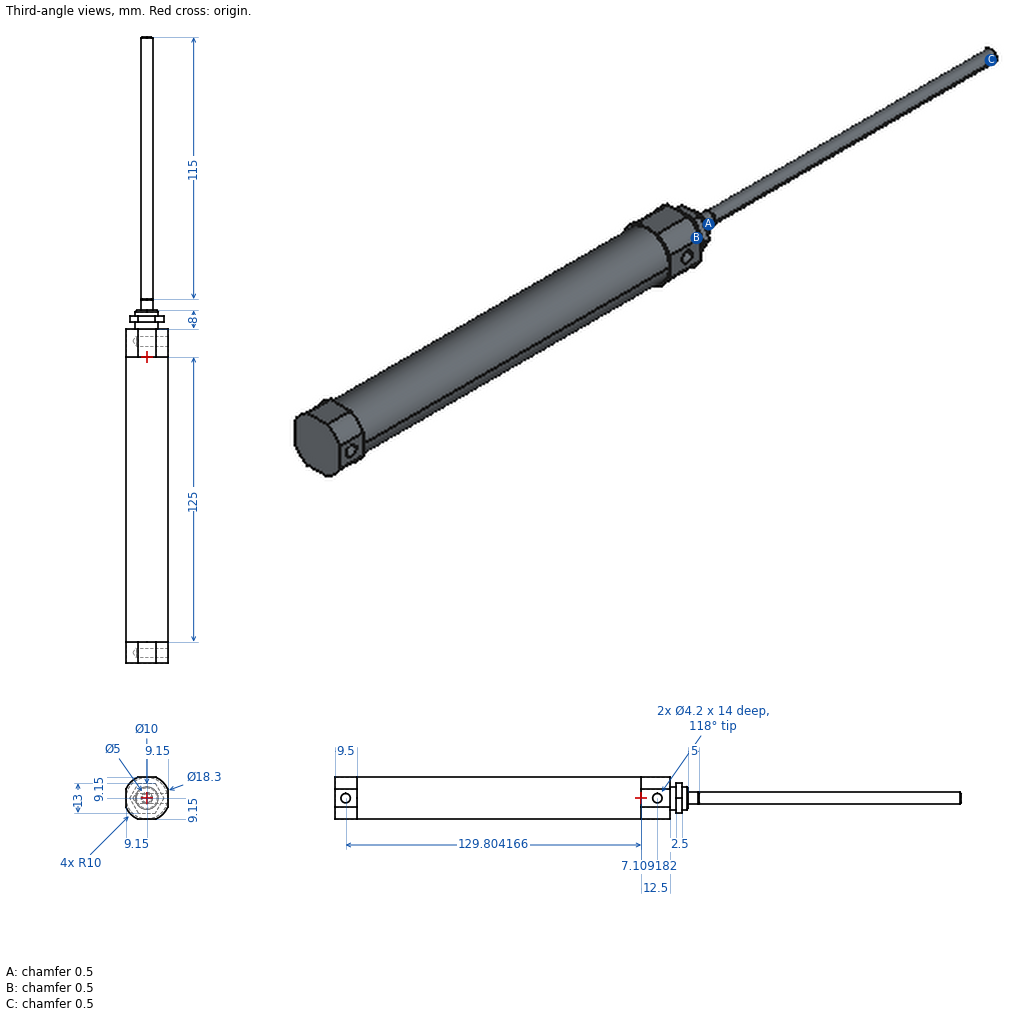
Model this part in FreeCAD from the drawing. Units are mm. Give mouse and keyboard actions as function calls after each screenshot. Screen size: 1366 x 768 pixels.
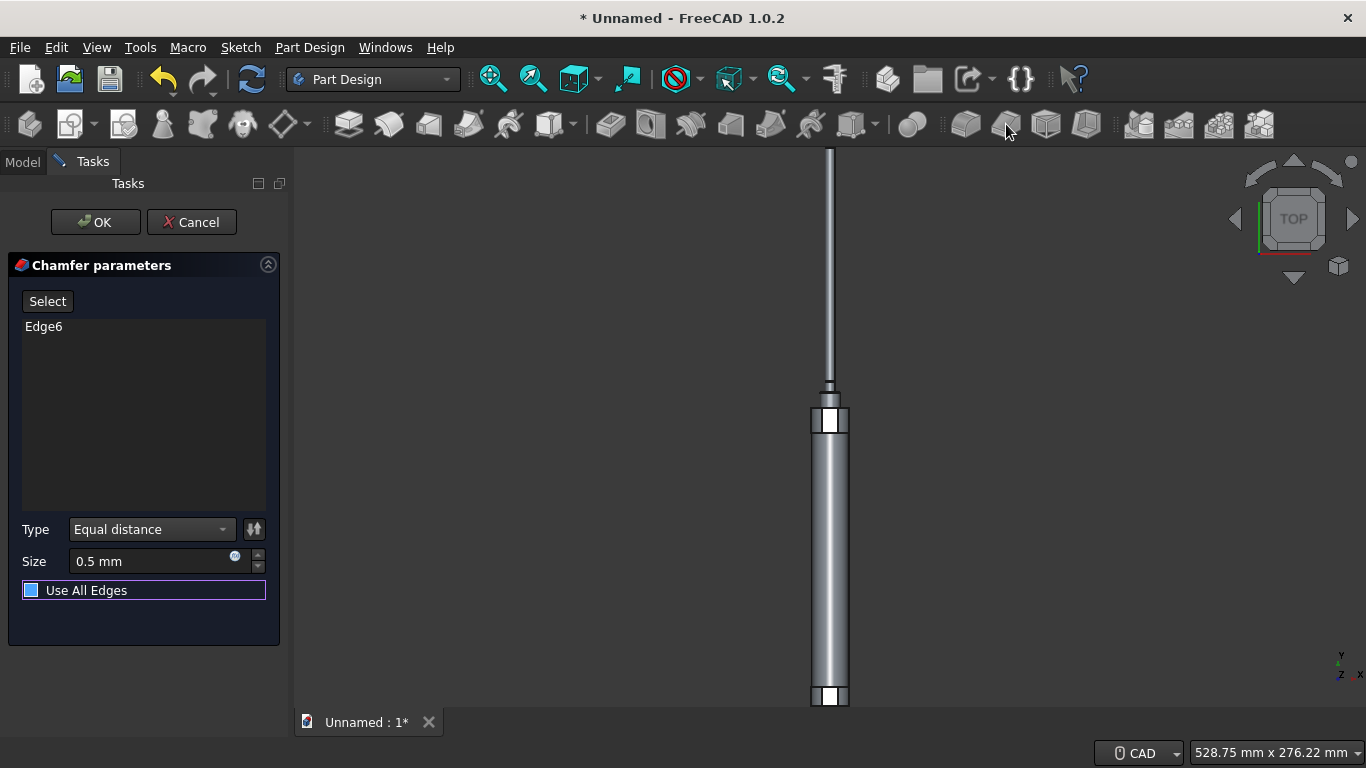
click(96, 222)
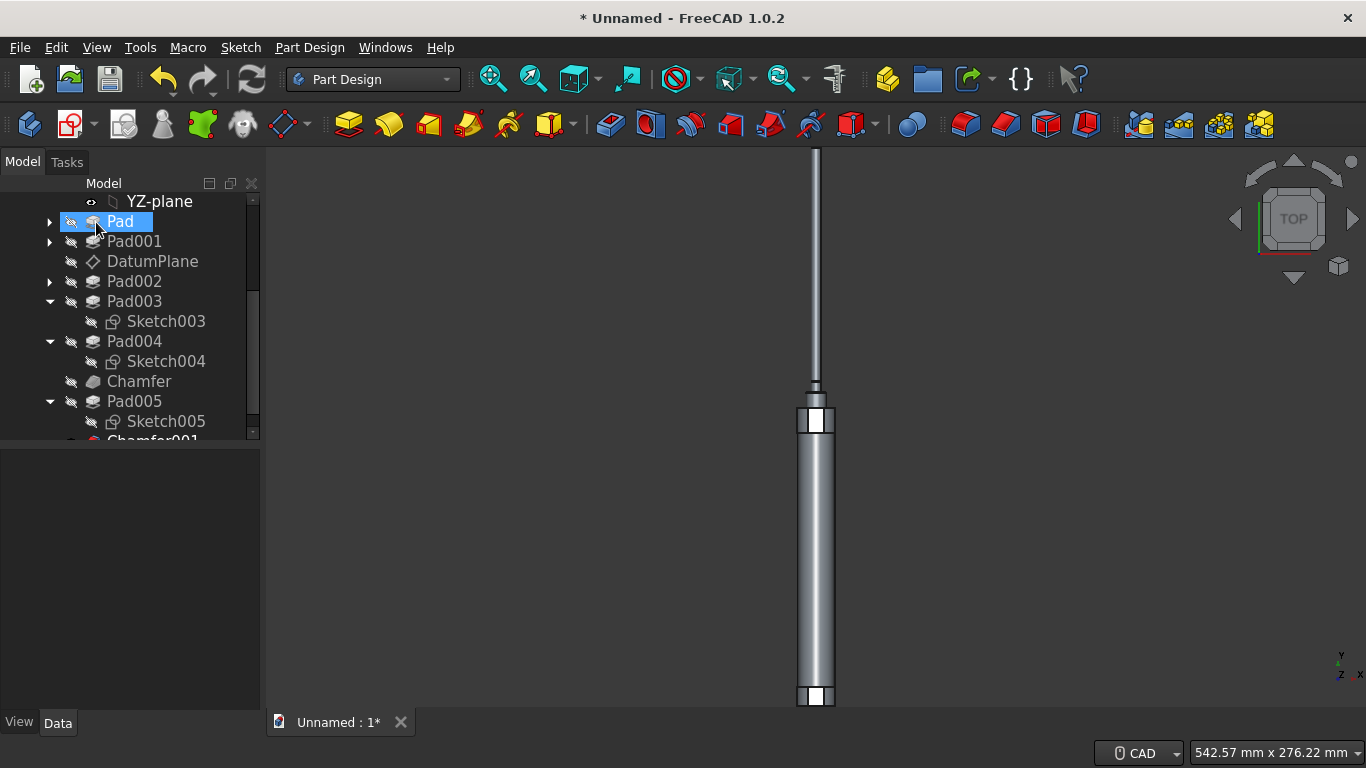
scroll(160, 317, down, 3)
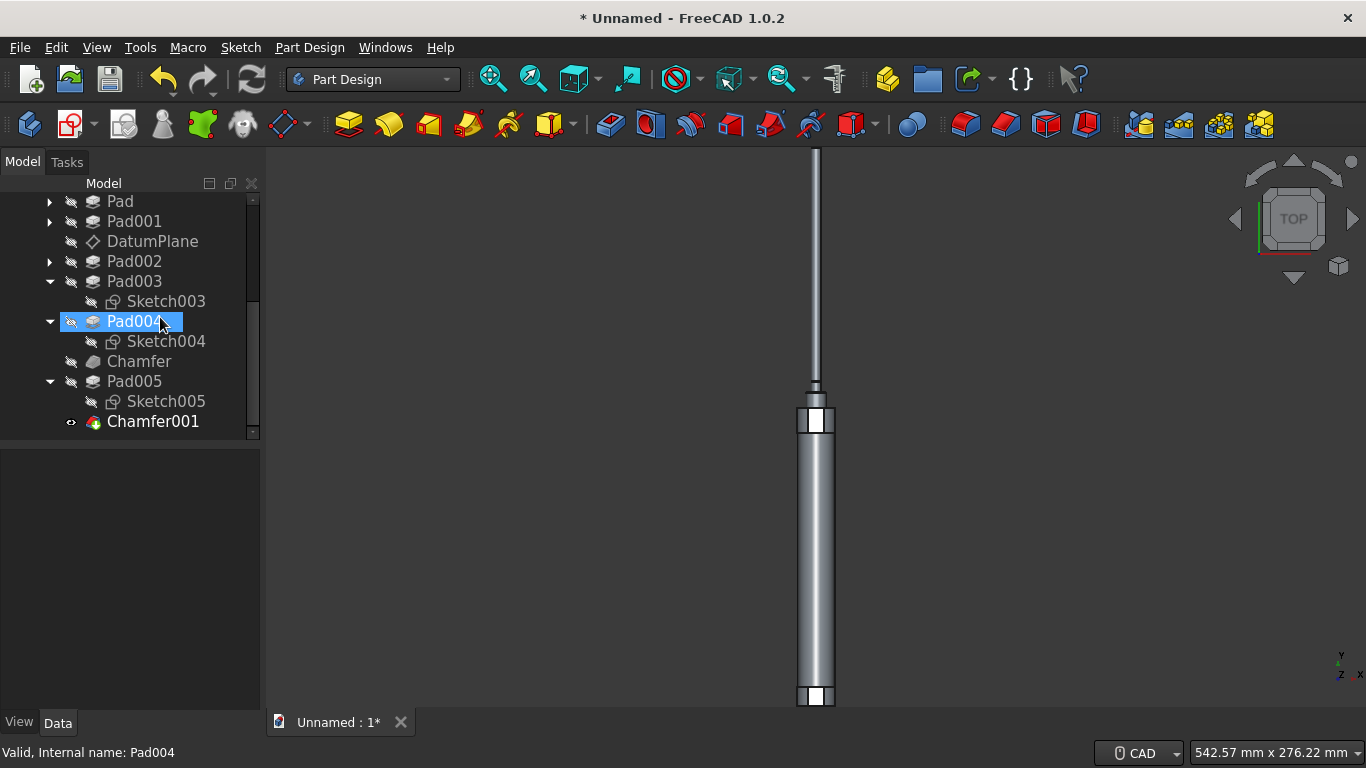
scroll(140, 317, up, 15)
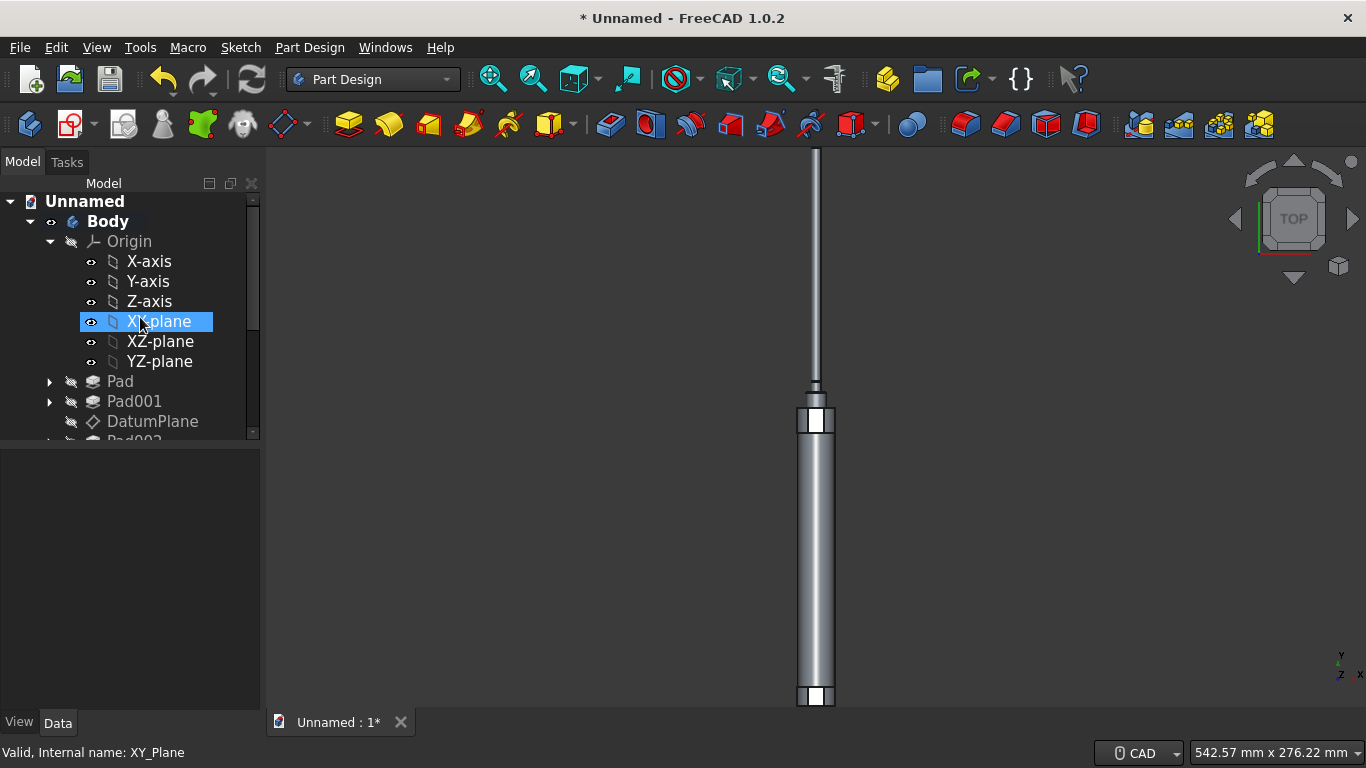
click(136, 342)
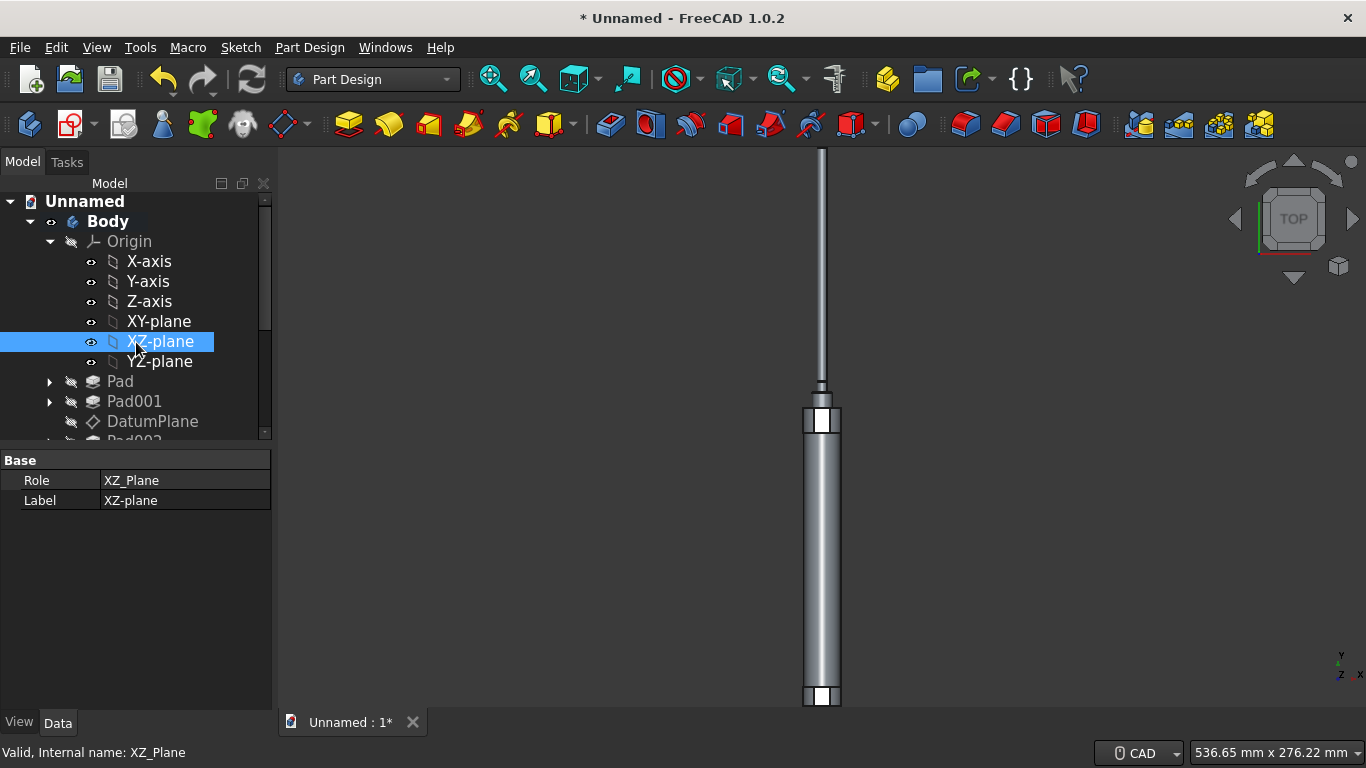
click(284, 124)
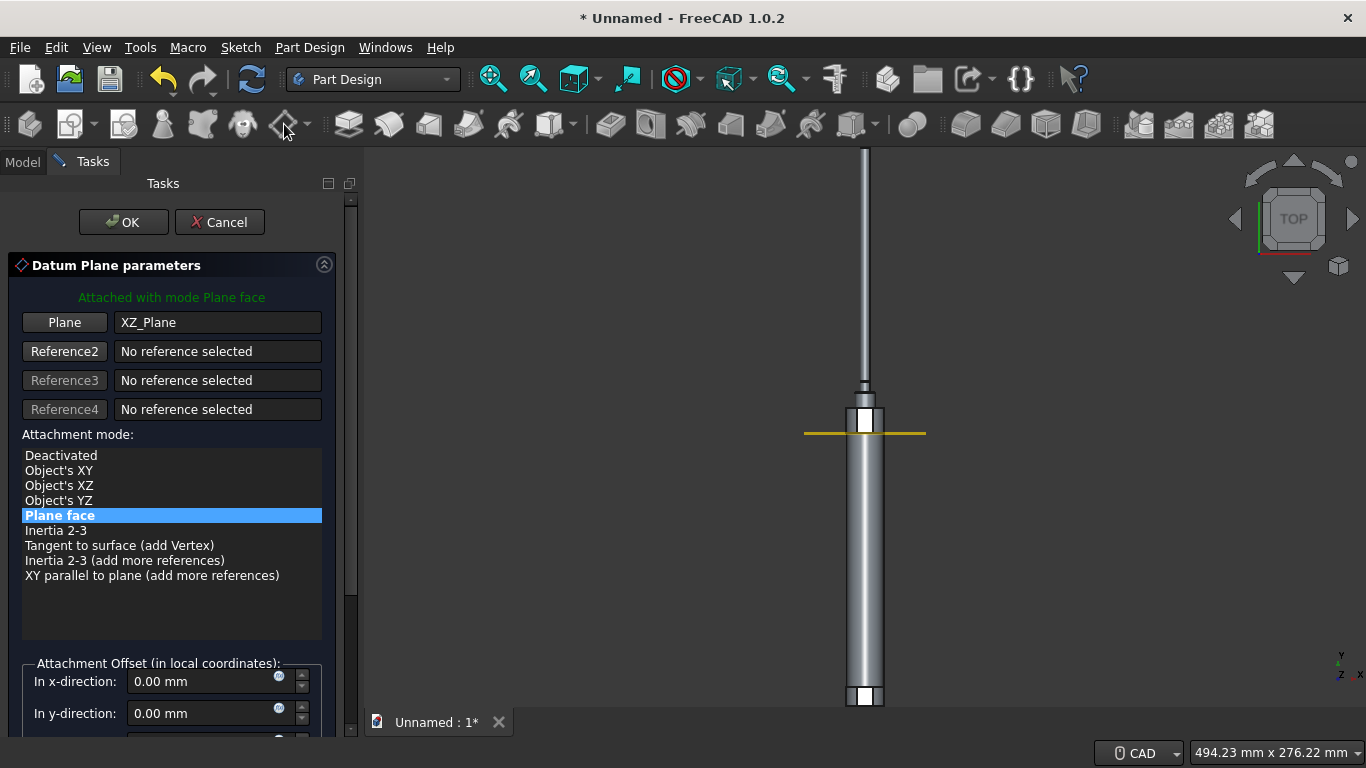
scroll(351, 464, down, 2)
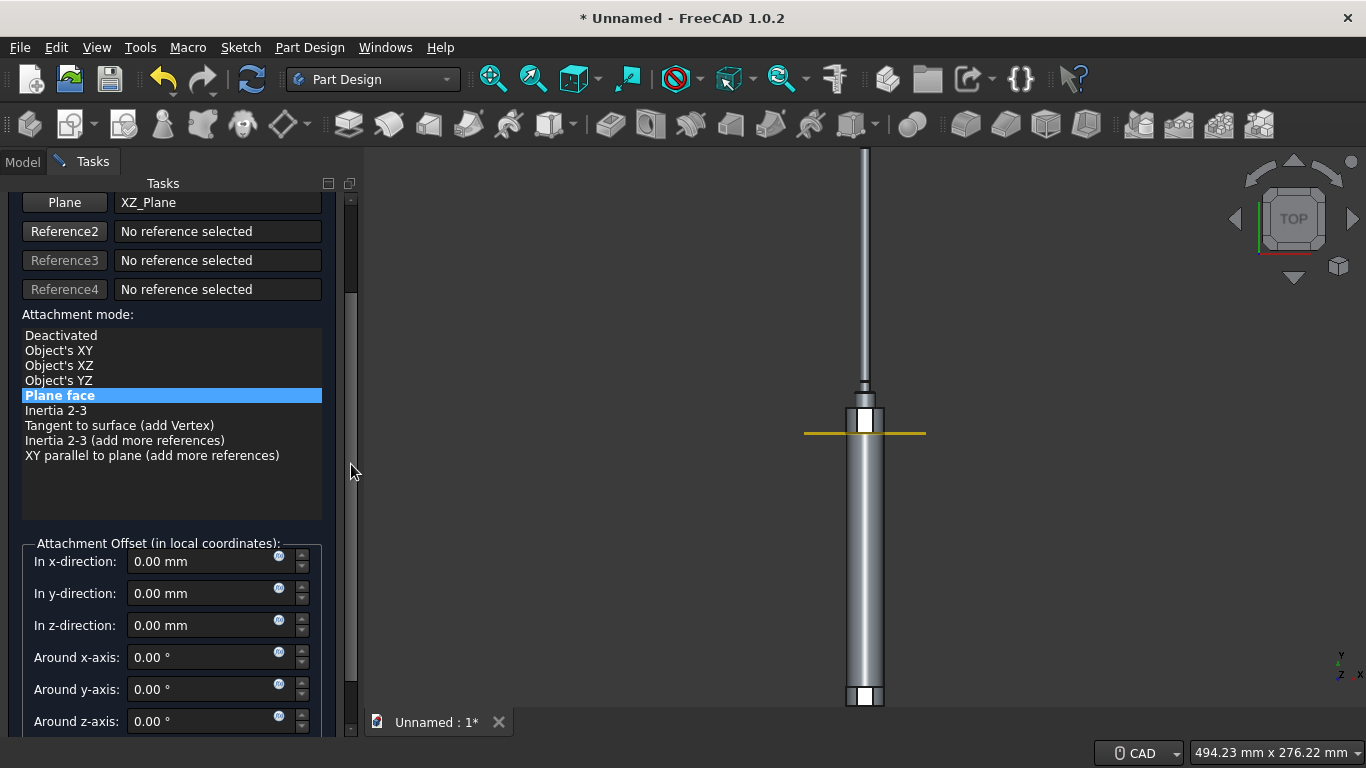
triple_click(210, 625)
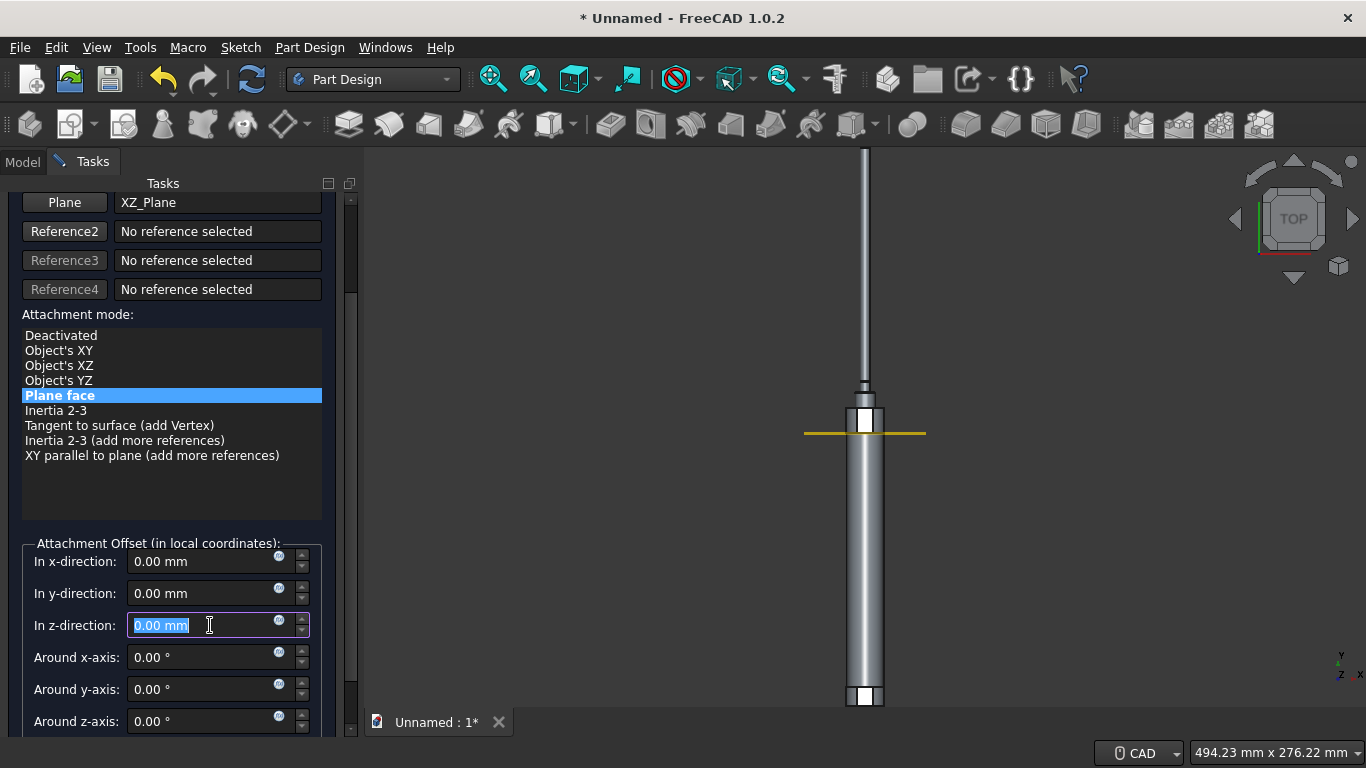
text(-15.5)
key(Tab)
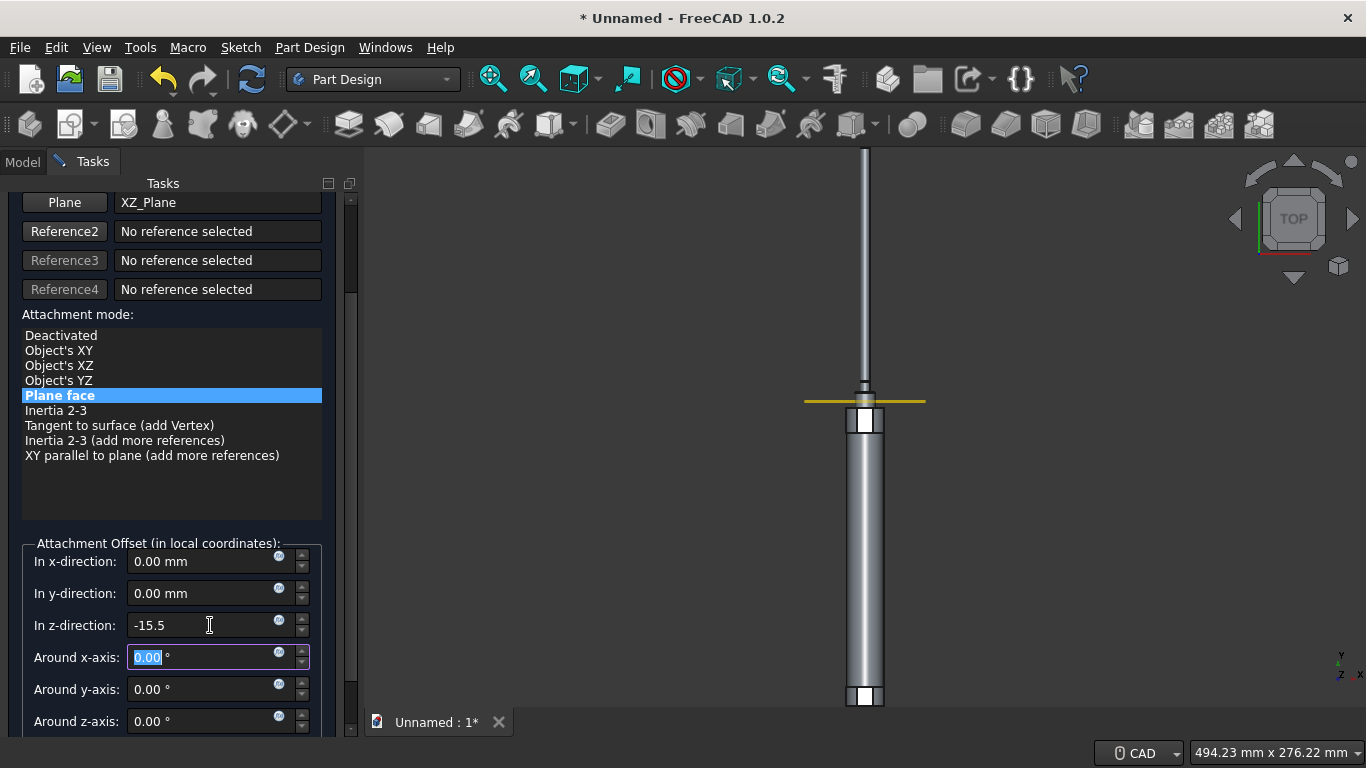
scroll(351, 464, up, 3)